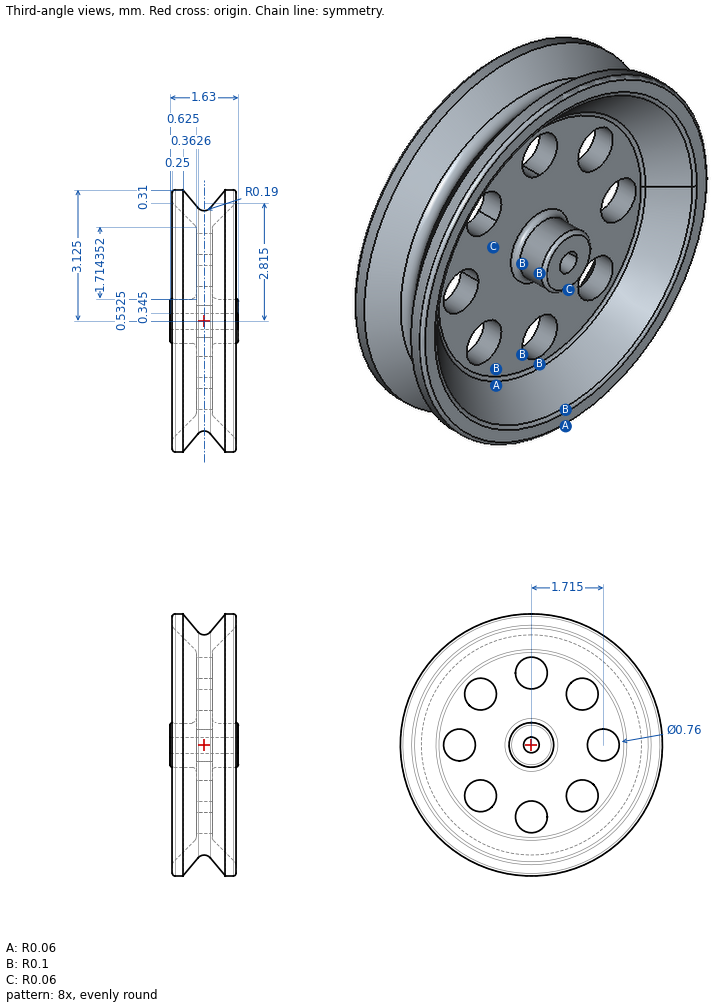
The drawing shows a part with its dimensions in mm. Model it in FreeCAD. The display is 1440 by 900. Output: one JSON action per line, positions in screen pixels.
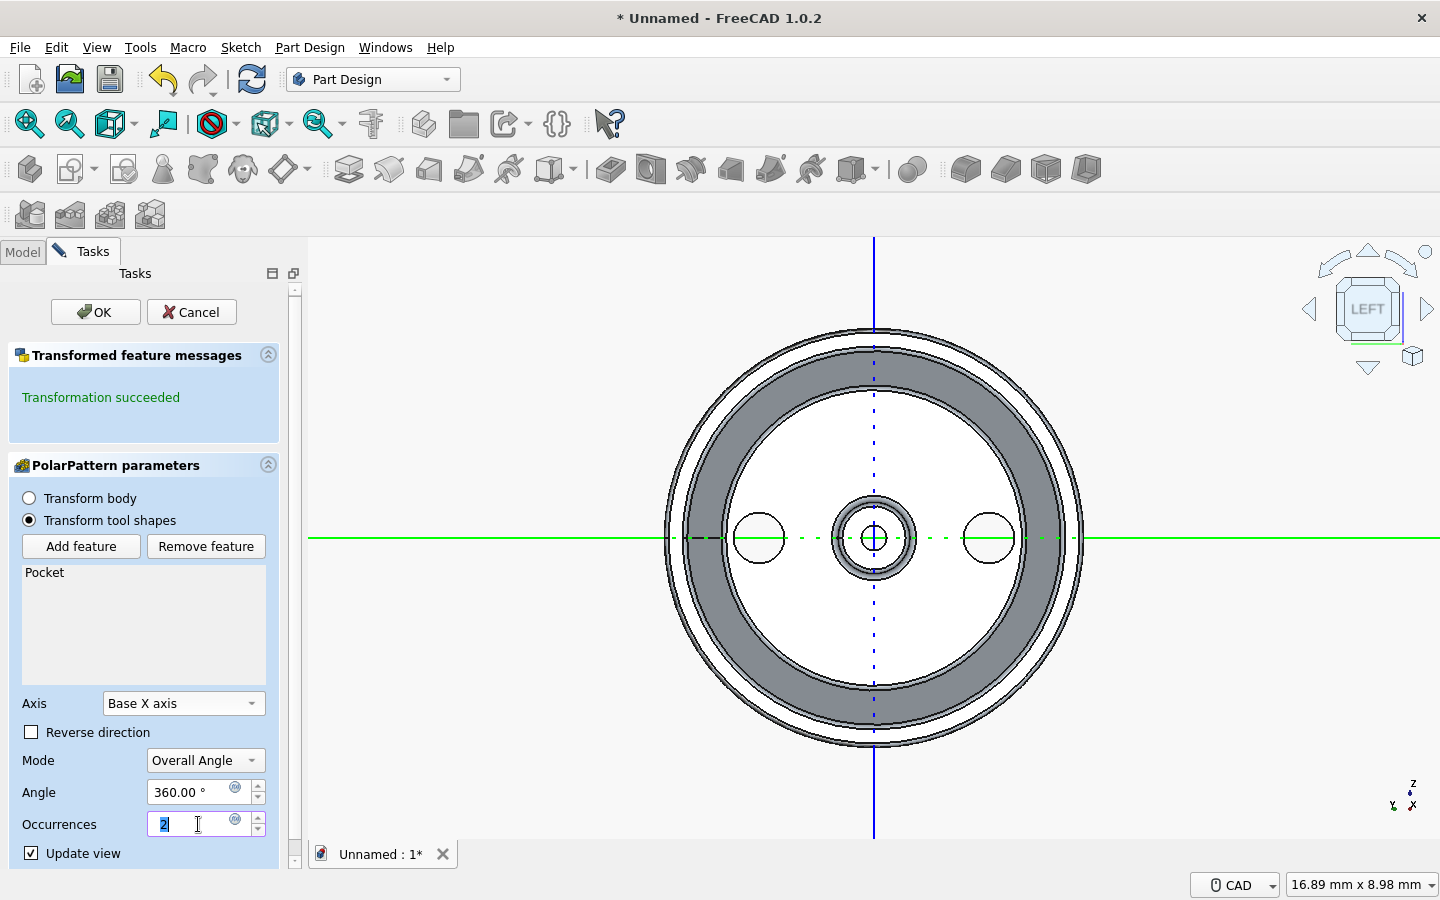
{"action": "type", "text": "8"}
{"action": "key", "text": "Tab"}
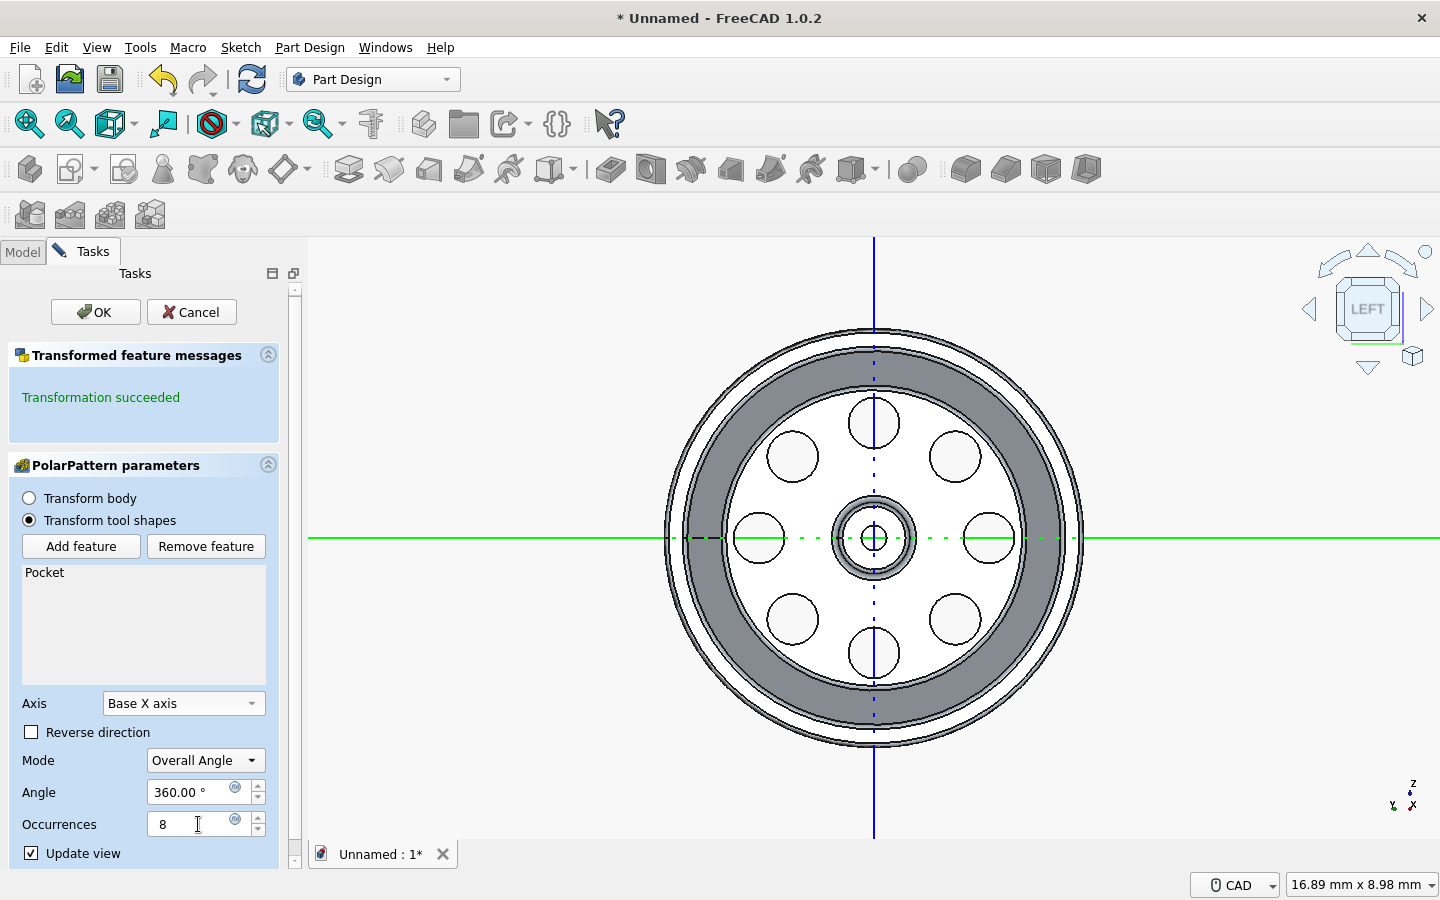
{"action": "left_click", "coordinate": [96, 312]}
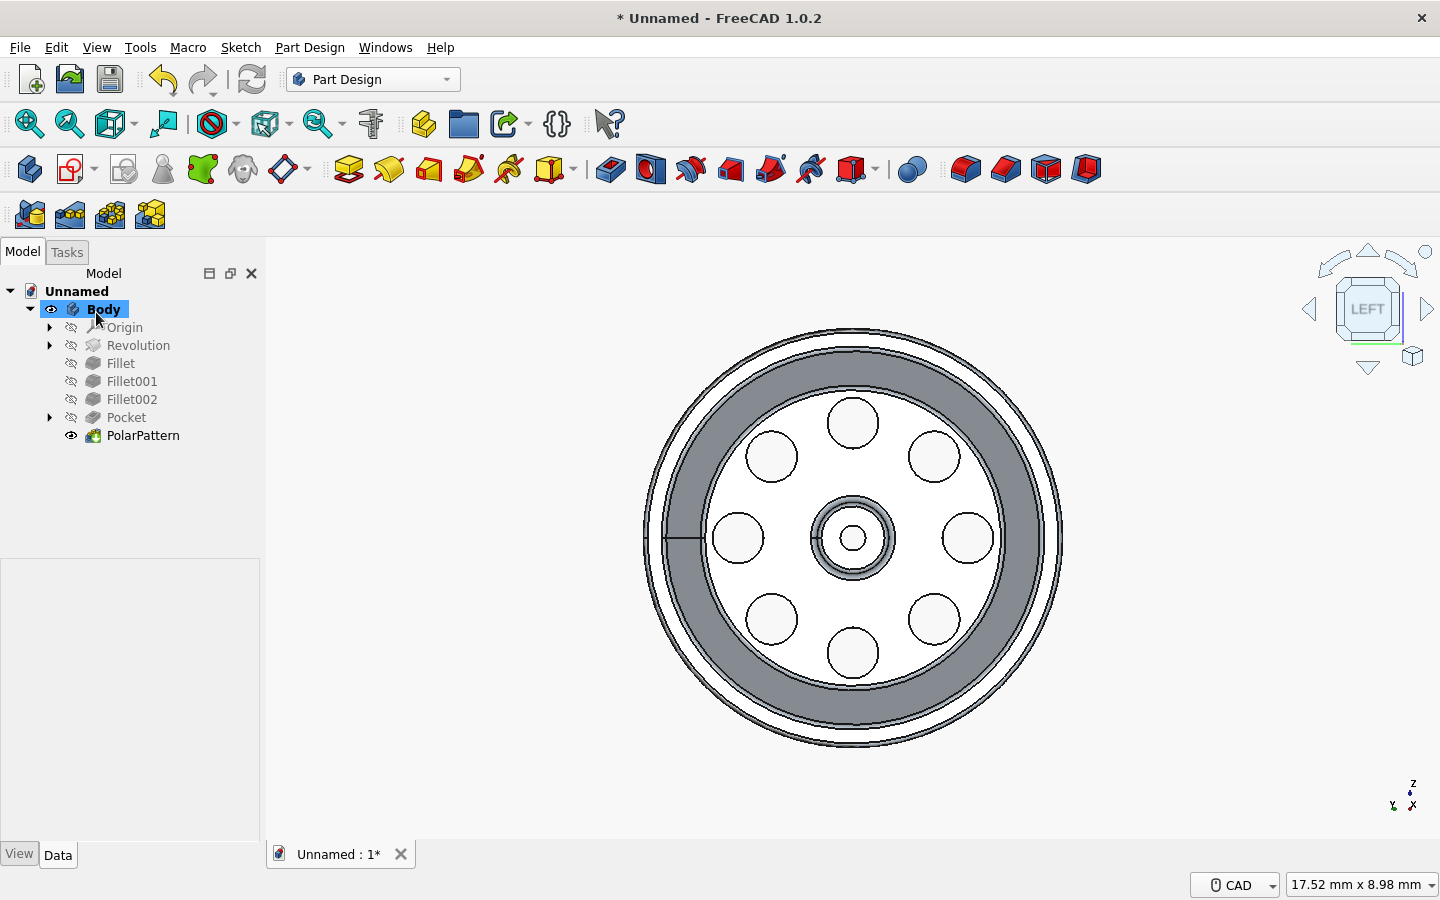
{"action": "key", "text": "0"}